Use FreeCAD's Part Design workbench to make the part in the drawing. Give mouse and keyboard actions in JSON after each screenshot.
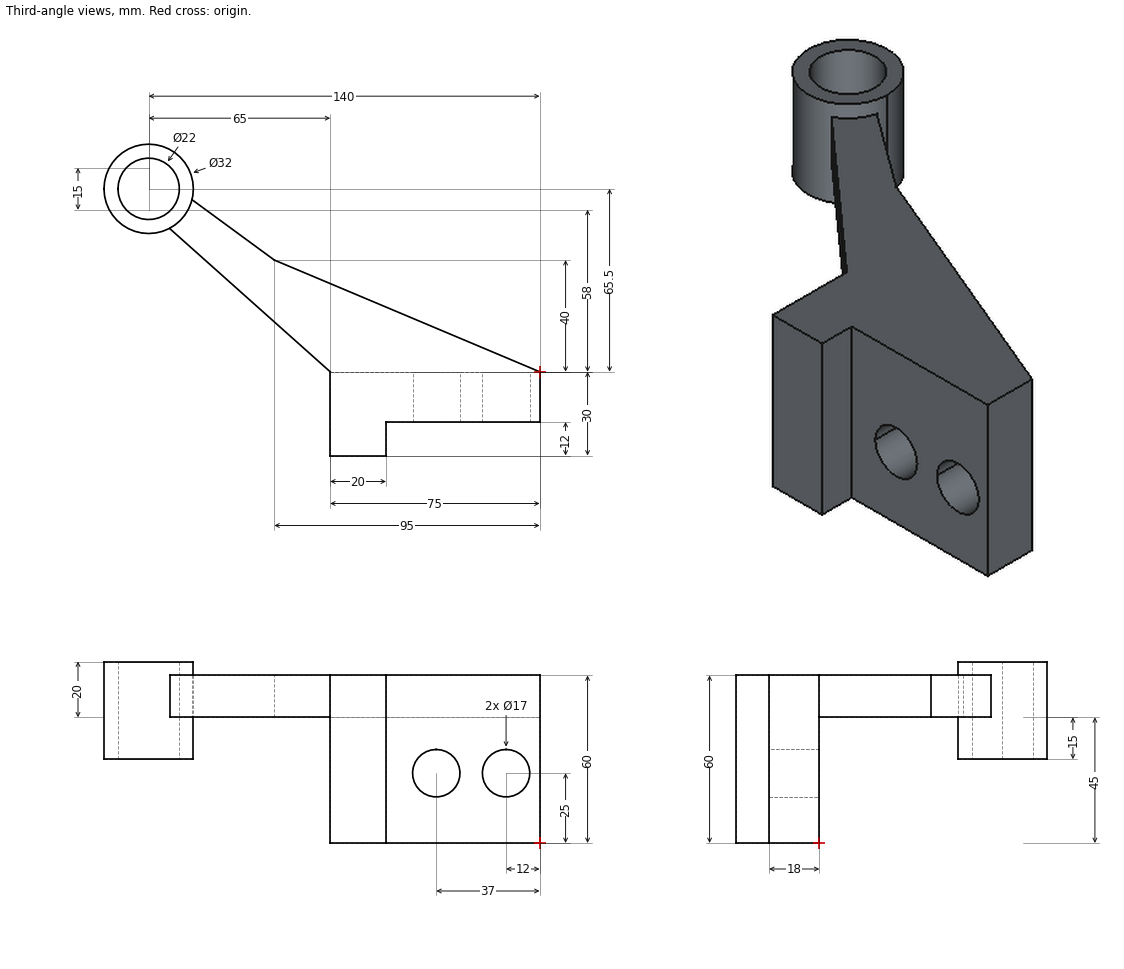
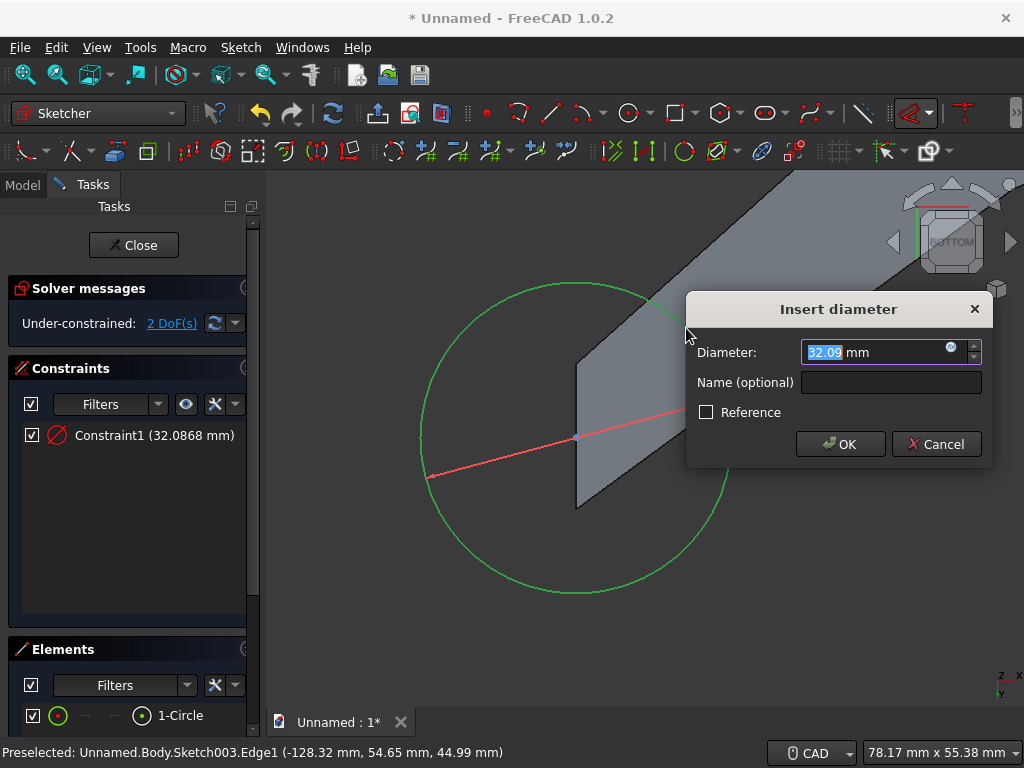
{"action": "type", "text": "32"}
{"action": "key", "text": "Return"}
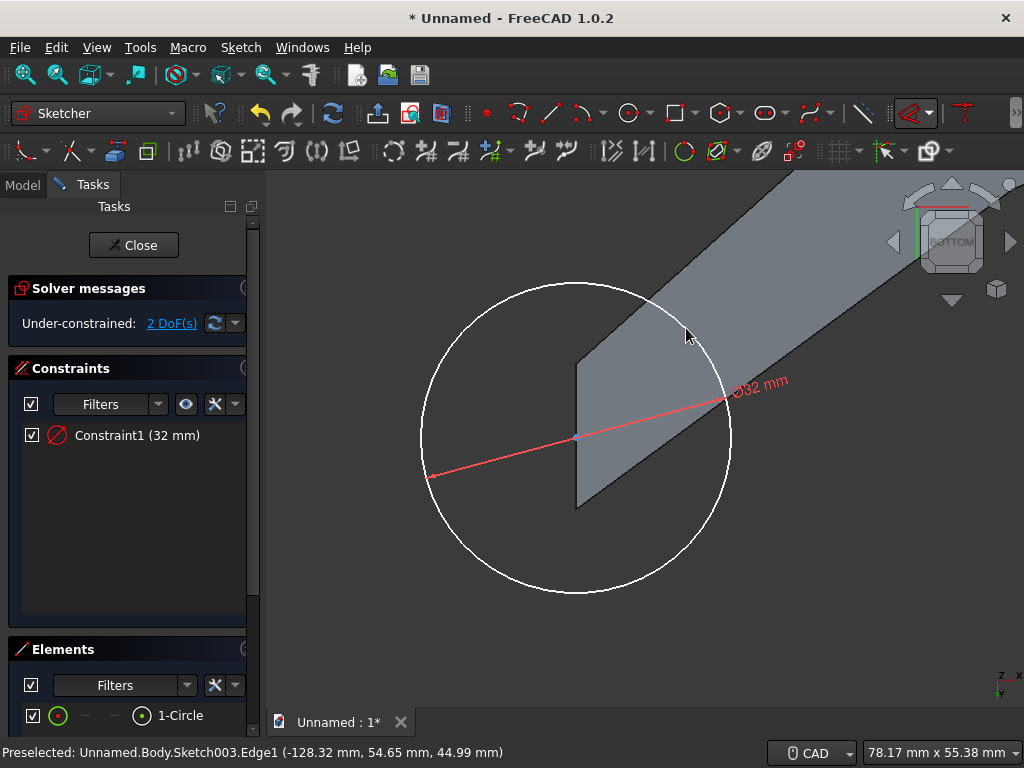
{"action": "left_click", "coordinate": [576, 438]}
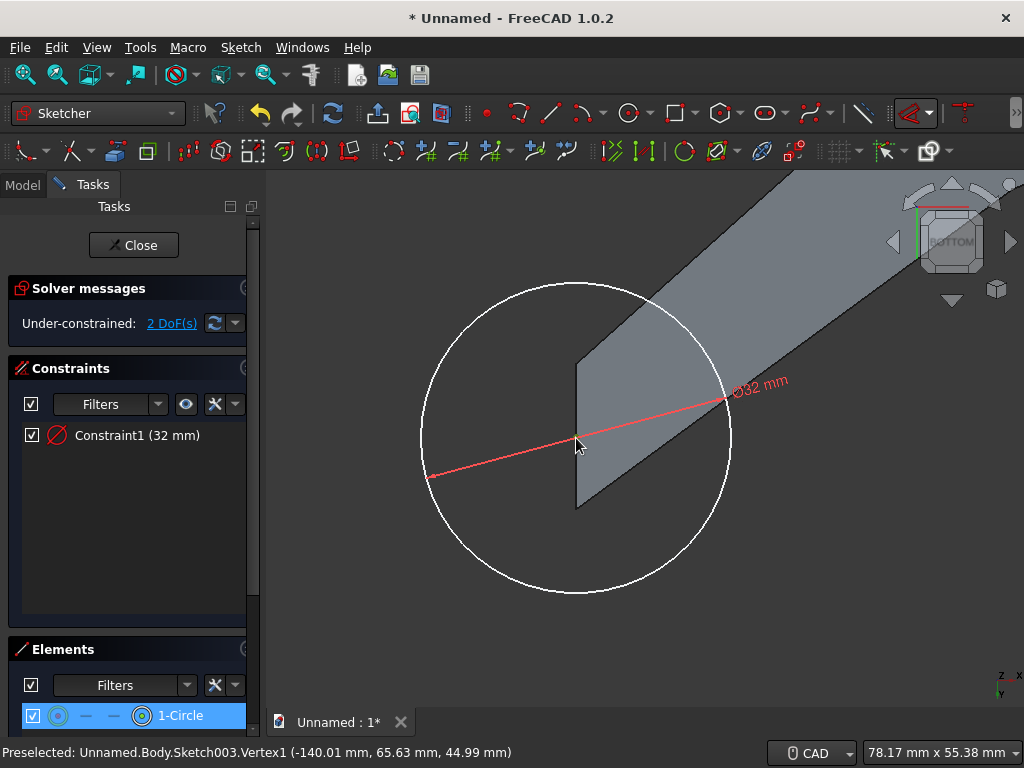
{"action": "left_click", "coordinate": [932, 114]}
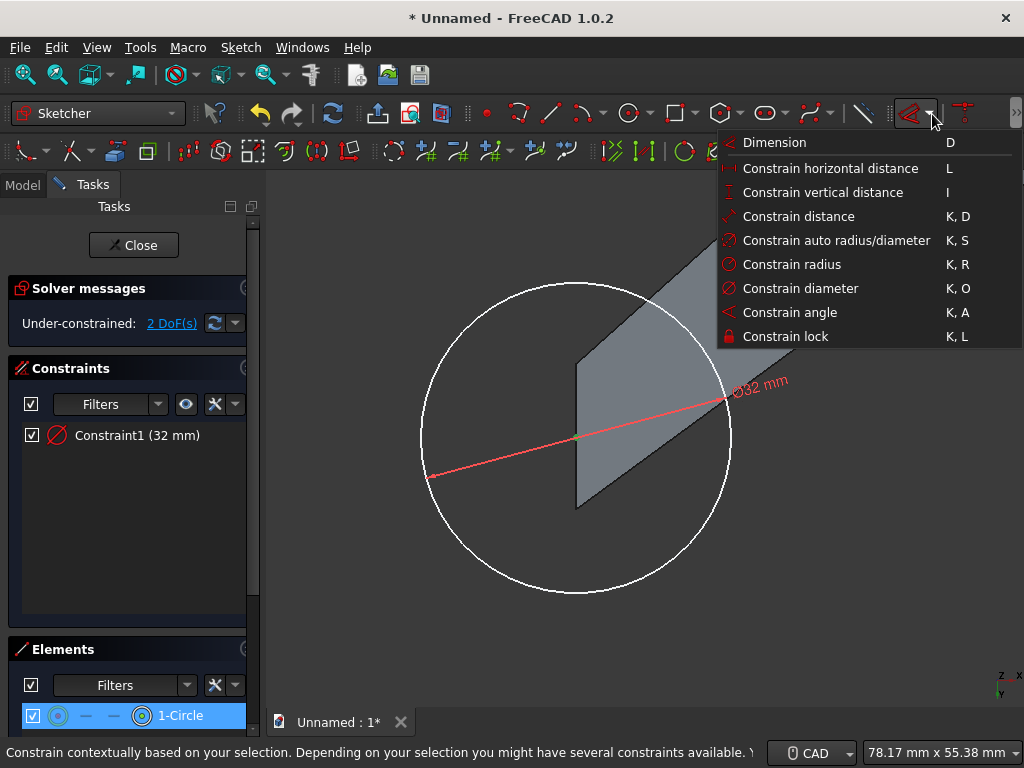
{"action": "left_click", "coordinate": [870, 168]}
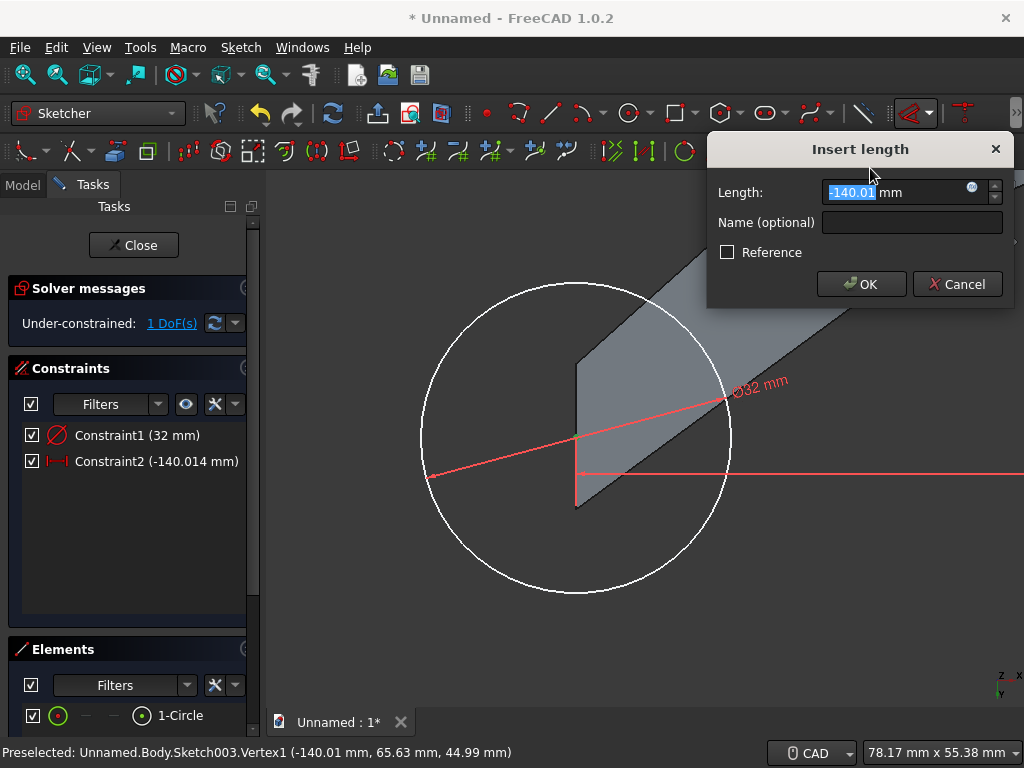
{"action": "type", "text": "-140"}
{"action": "key", "text": "Return"}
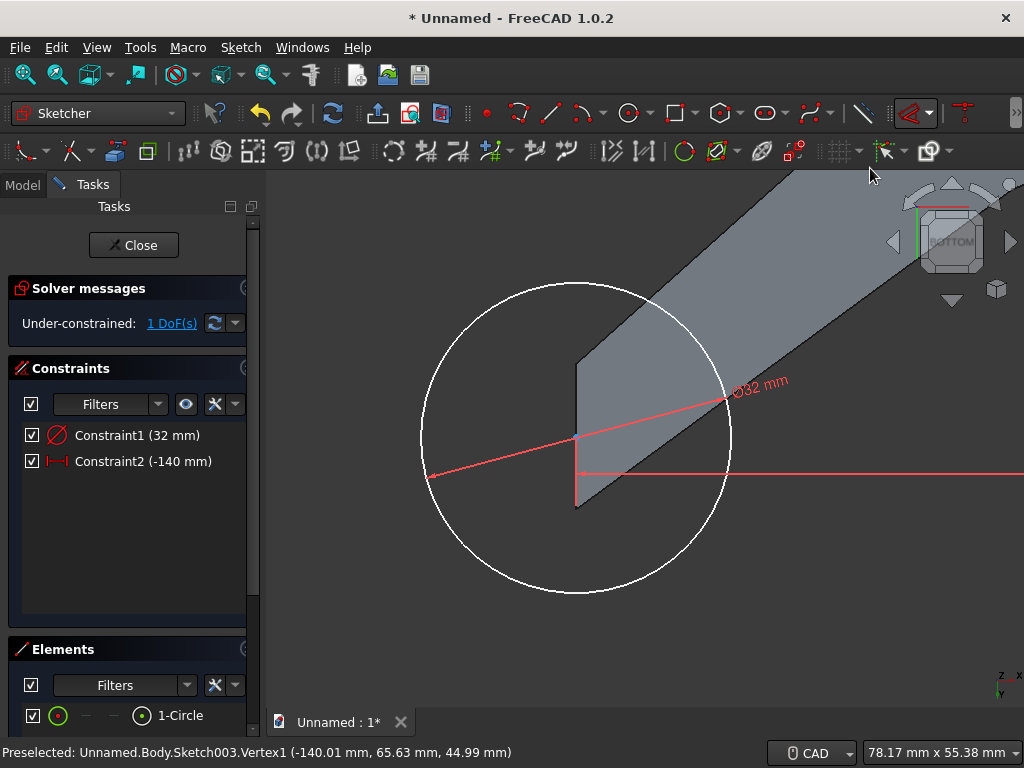
{"action": "left_click", "coordinate": [576, 438]}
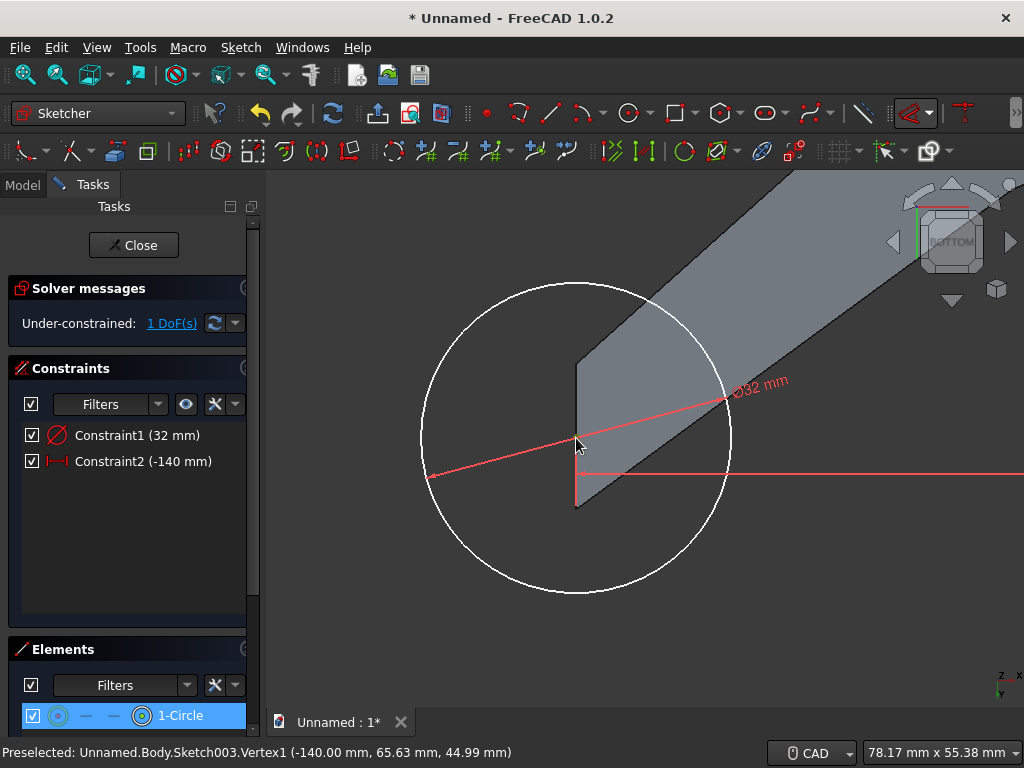
{"action": "left_click", "coordinate": [932, 114]}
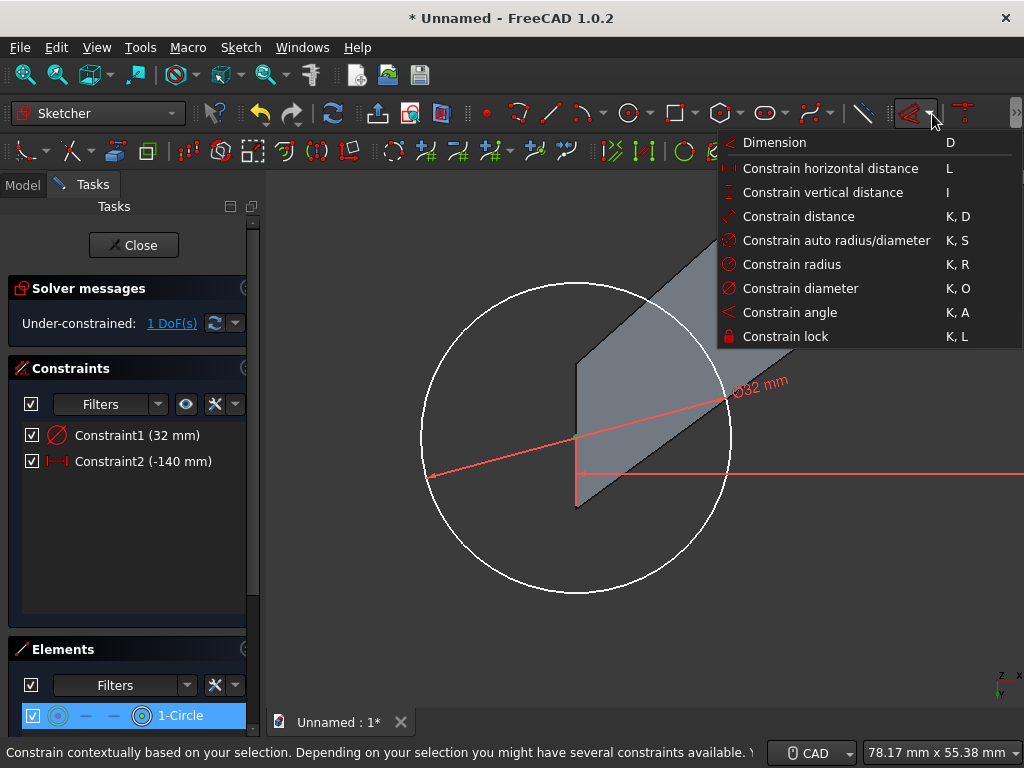
{"action": "left_click", "coordinate": [870, 192]}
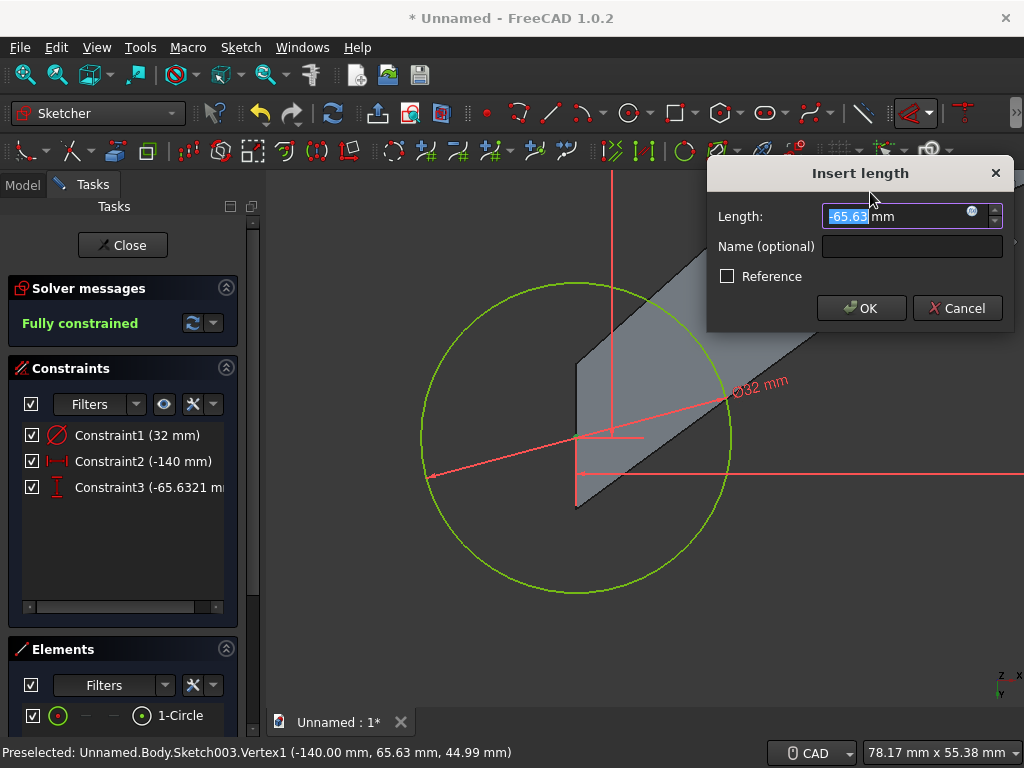
{"action": "type", "text": "-65.5"}
{"action": "key", "text": "Return"}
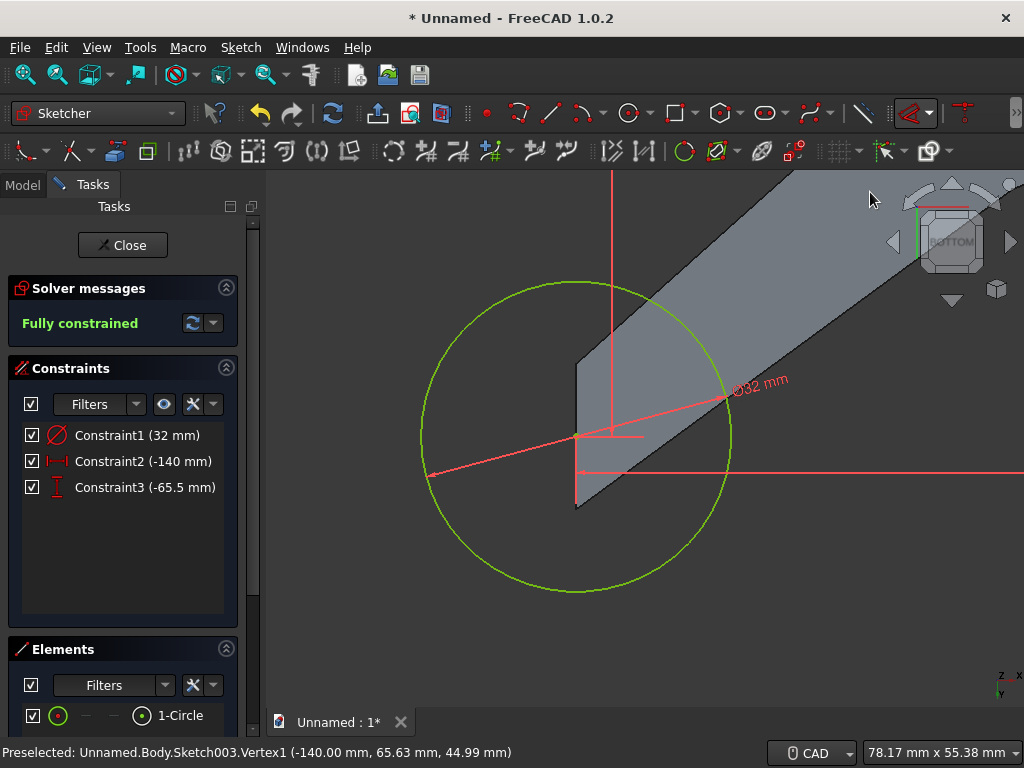
{"action": "left_click", "coordinate": [123, 245]}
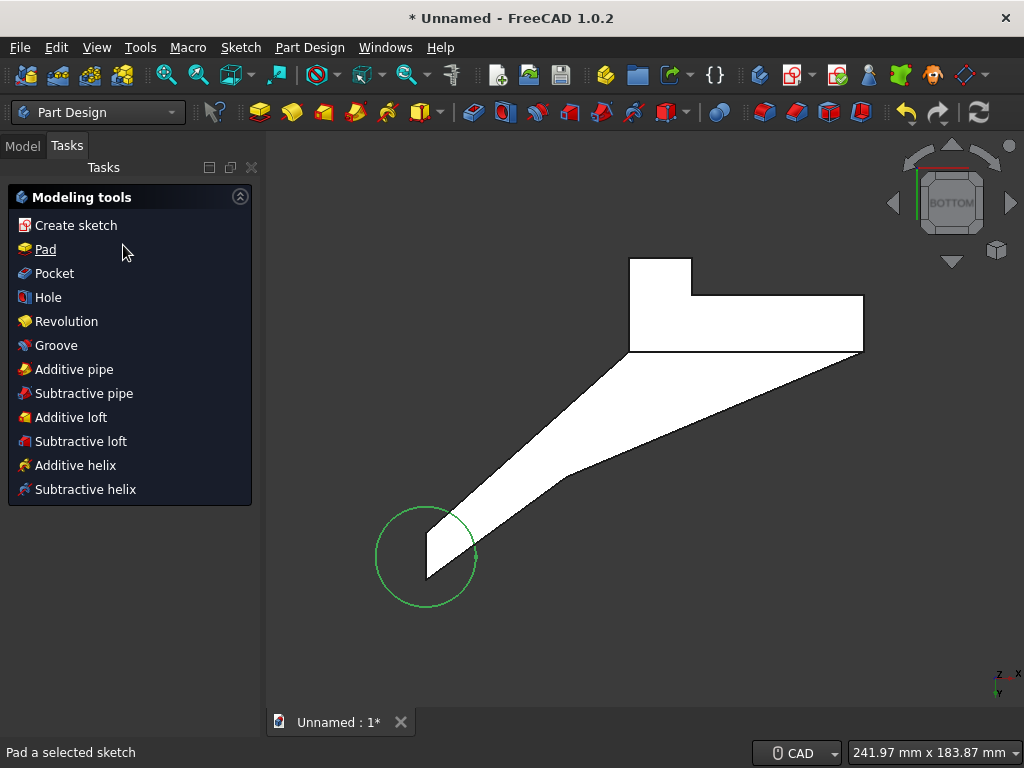
{"action": "left_click", "coordinate": [260, 112]}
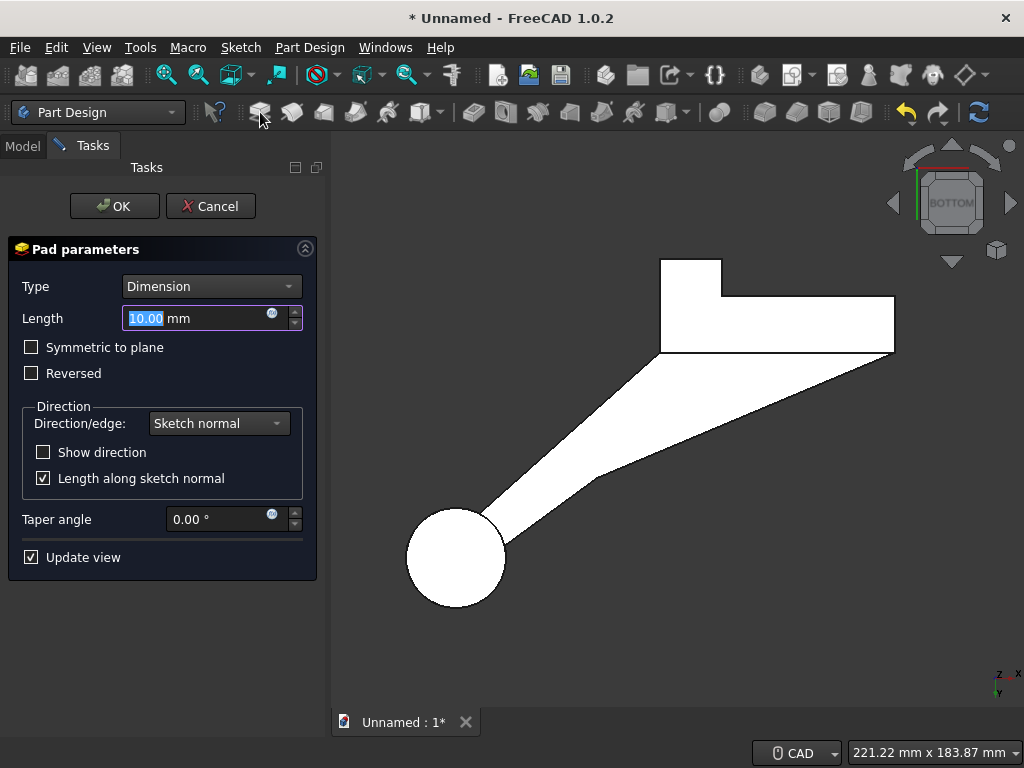
{"action": "type", "text": "20"}
{"action": "key", "text": "Tab"}